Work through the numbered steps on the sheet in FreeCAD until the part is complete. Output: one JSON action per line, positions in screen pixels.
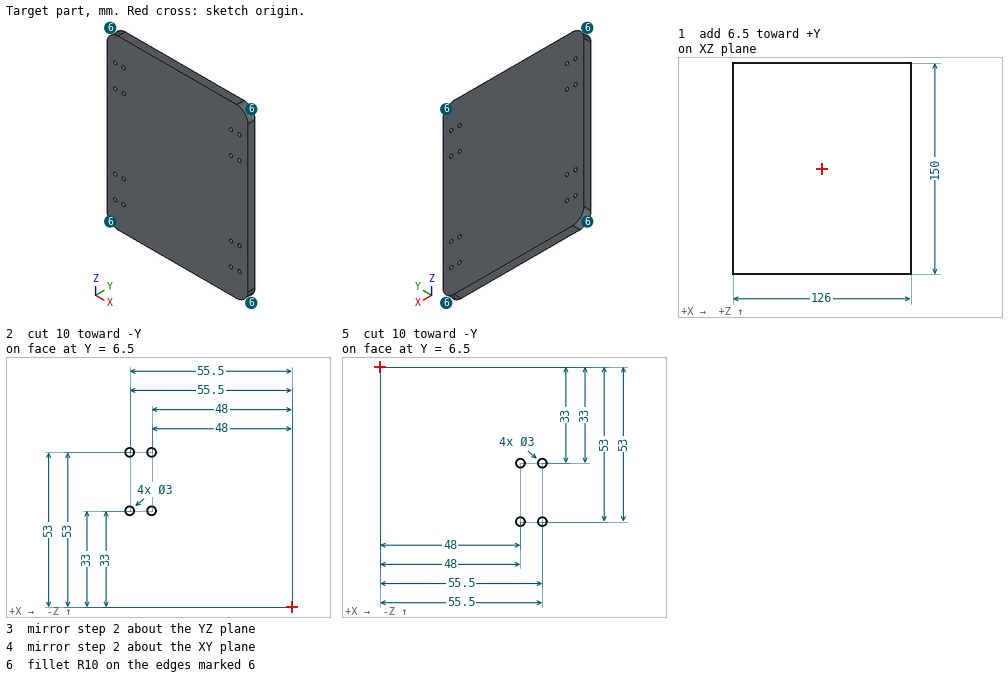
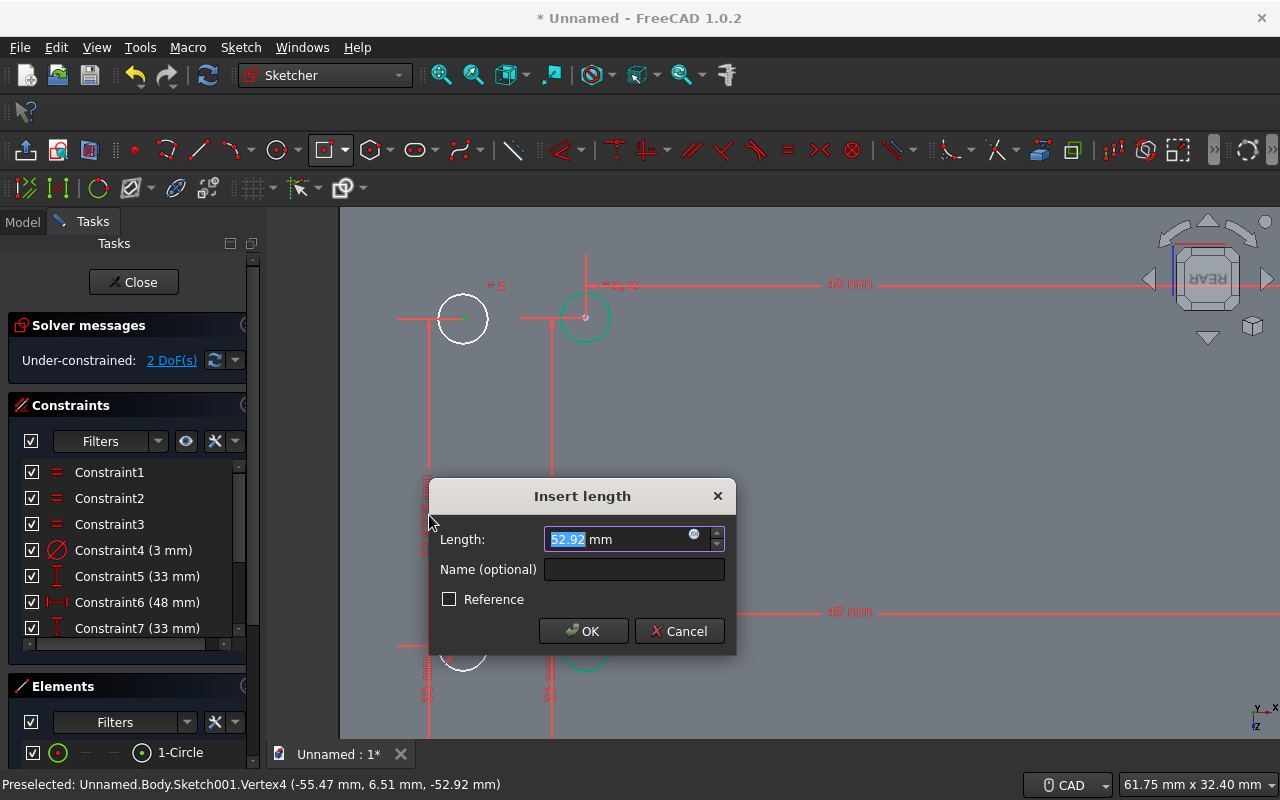
{"action": "type", "text": "53"}
{"action": "key", "text": "Return"}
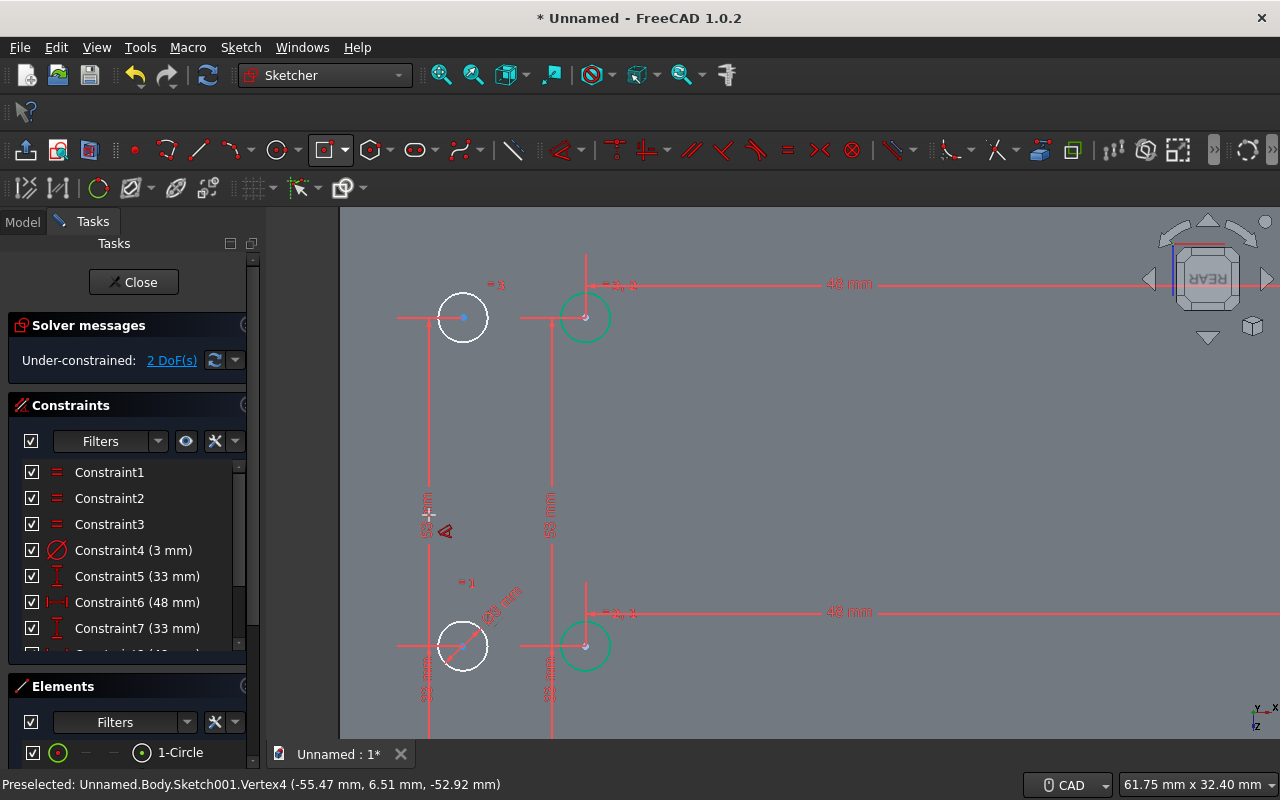
{"action": "left_click", "coordinate": [463, 646]}
{"action": "left_click", "coordinate": [639, 612]}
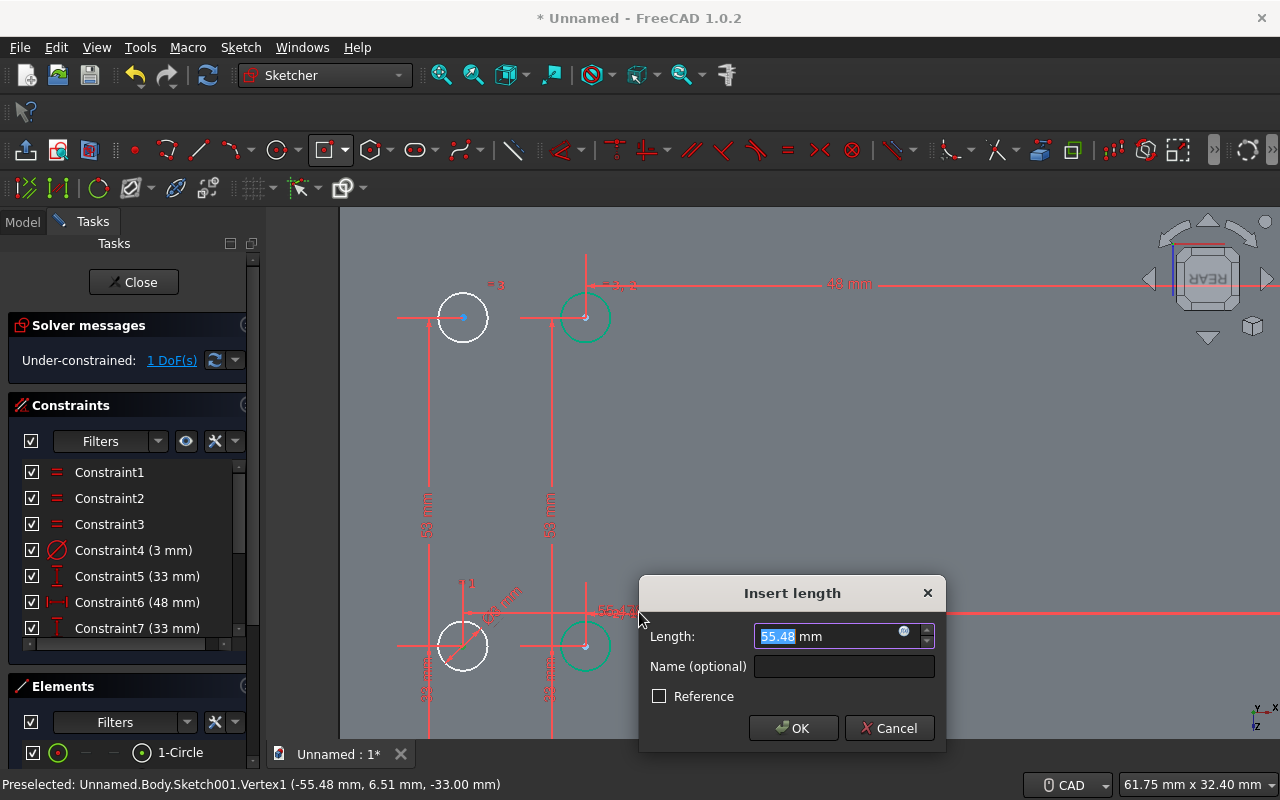
{"action": "type", "text": "55.5"}
{"action": "key", "text": "Return"}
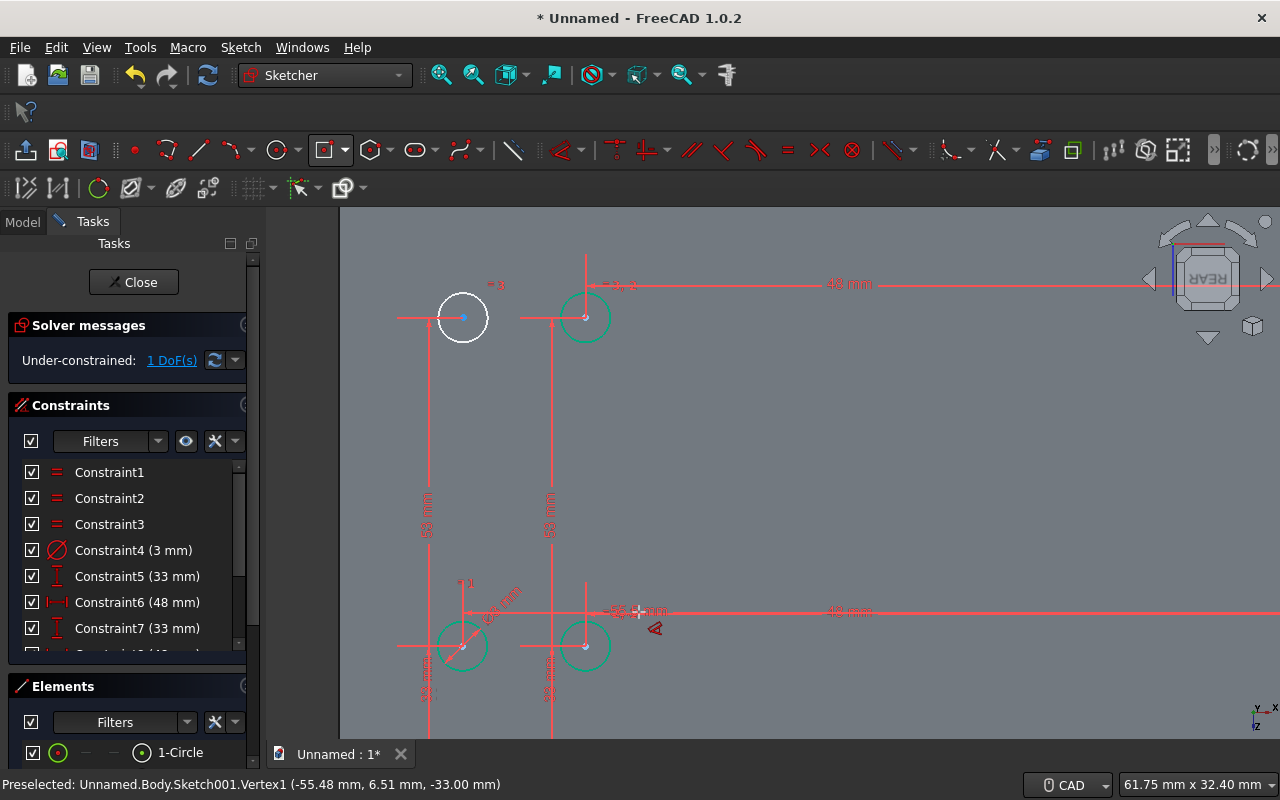
{"action": "left_click", "coordinate": [463, 318]}
{"action": "left_click", "coordinate": [639, 284]}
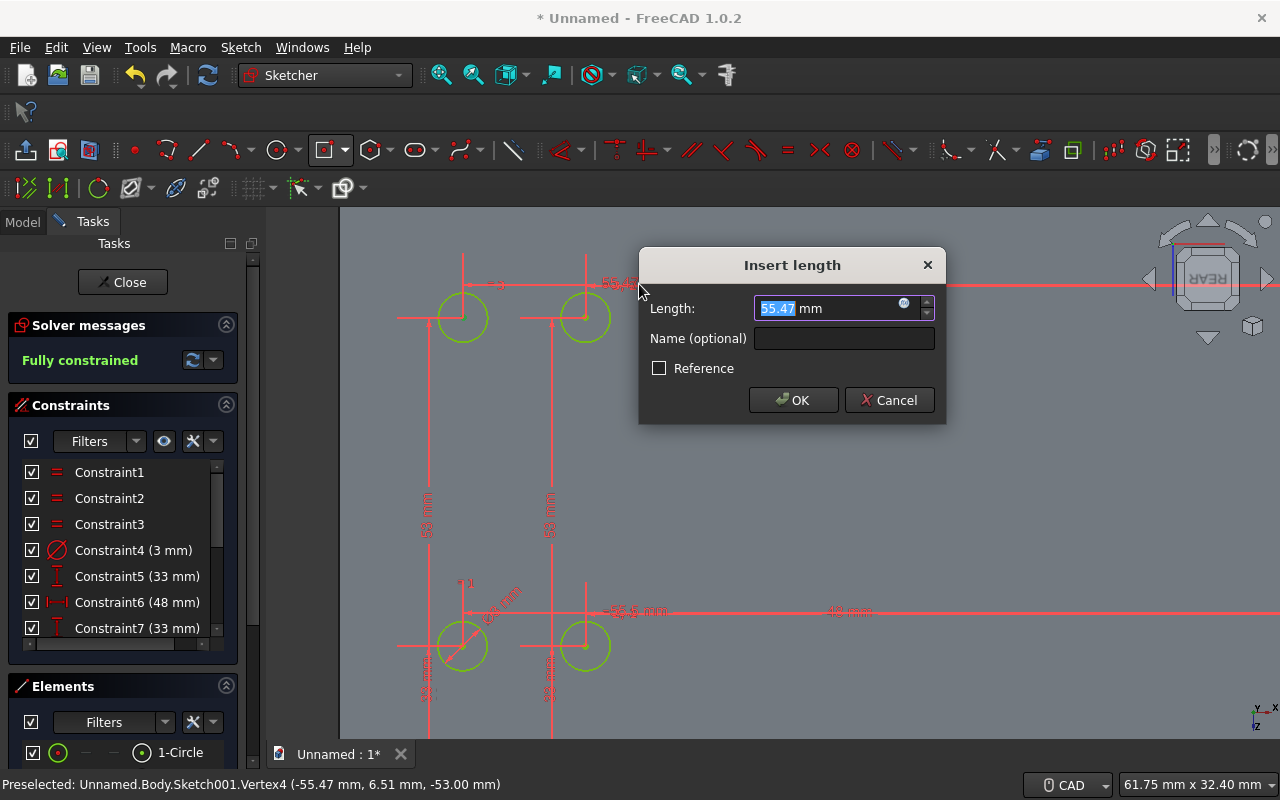
{"action": "type", "text": "55.5"}
{"action": "key", "text": "Return"}
{"action": "key", "text": "Escape"}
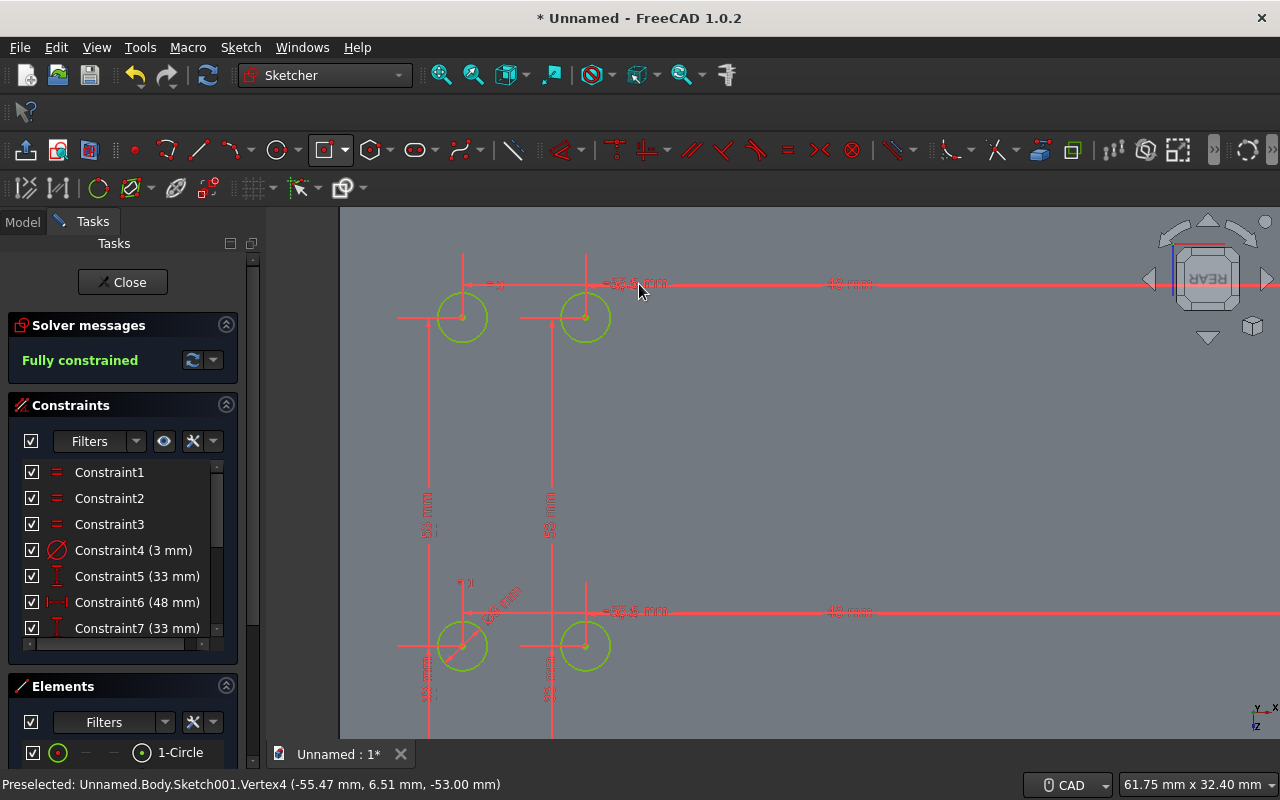
{"action": "left_click", "coordinate": [123, 282]}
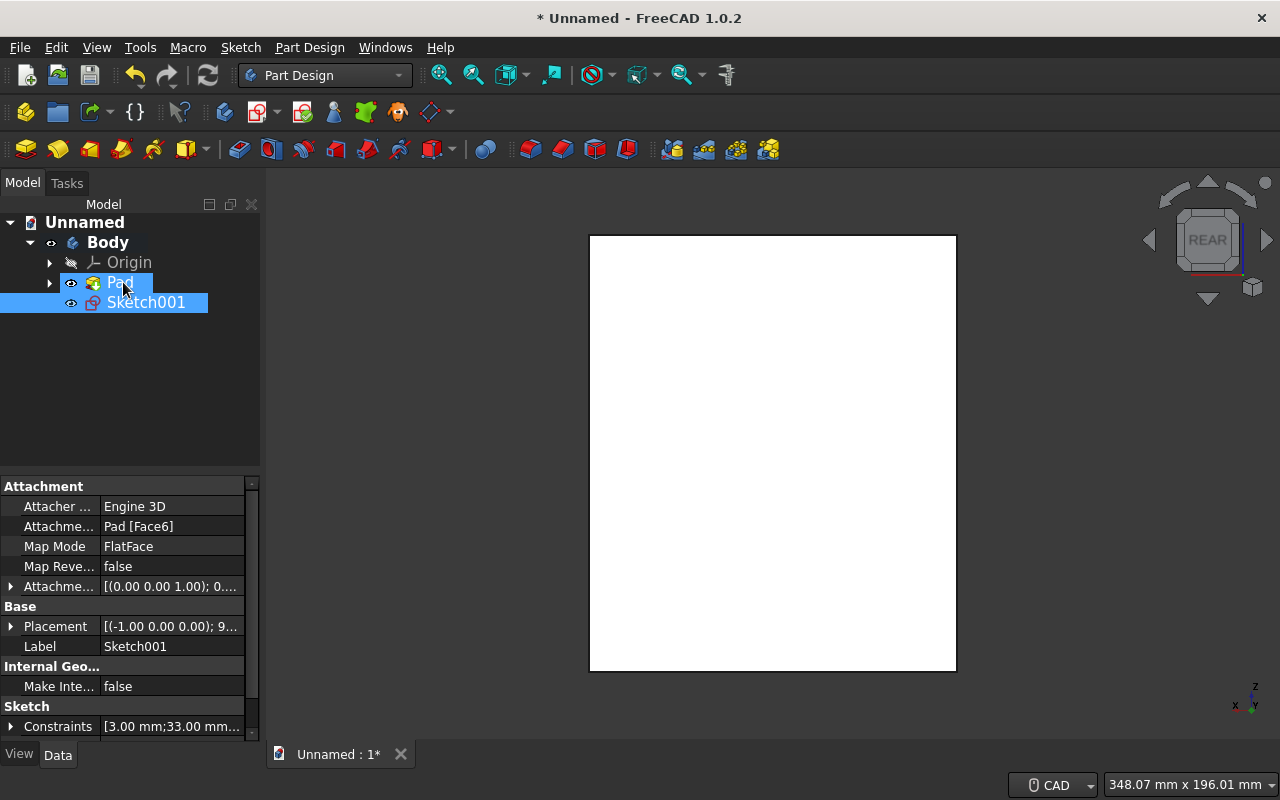
{"action": "left_click", "coordinate": [240, 150]}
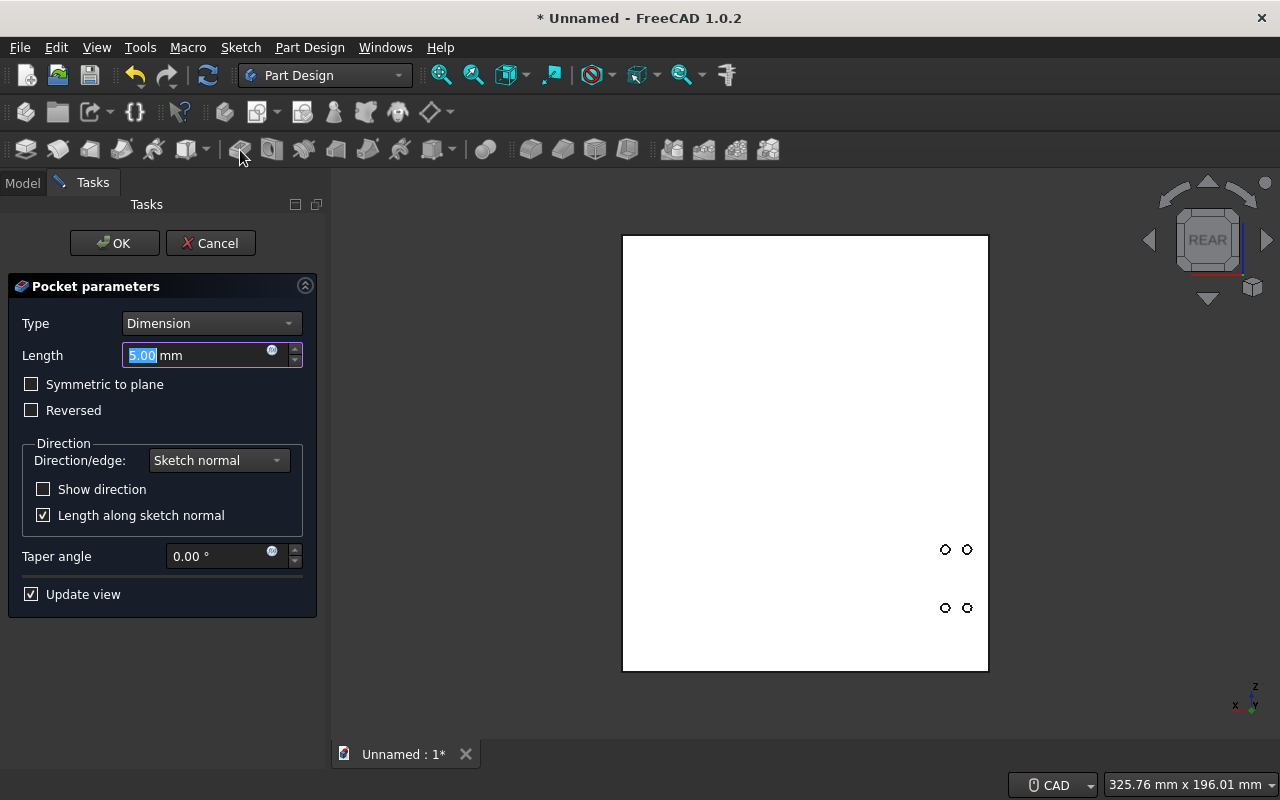
{"action": "type", "text": "10"}
{"action": "key", "text": "Tab"}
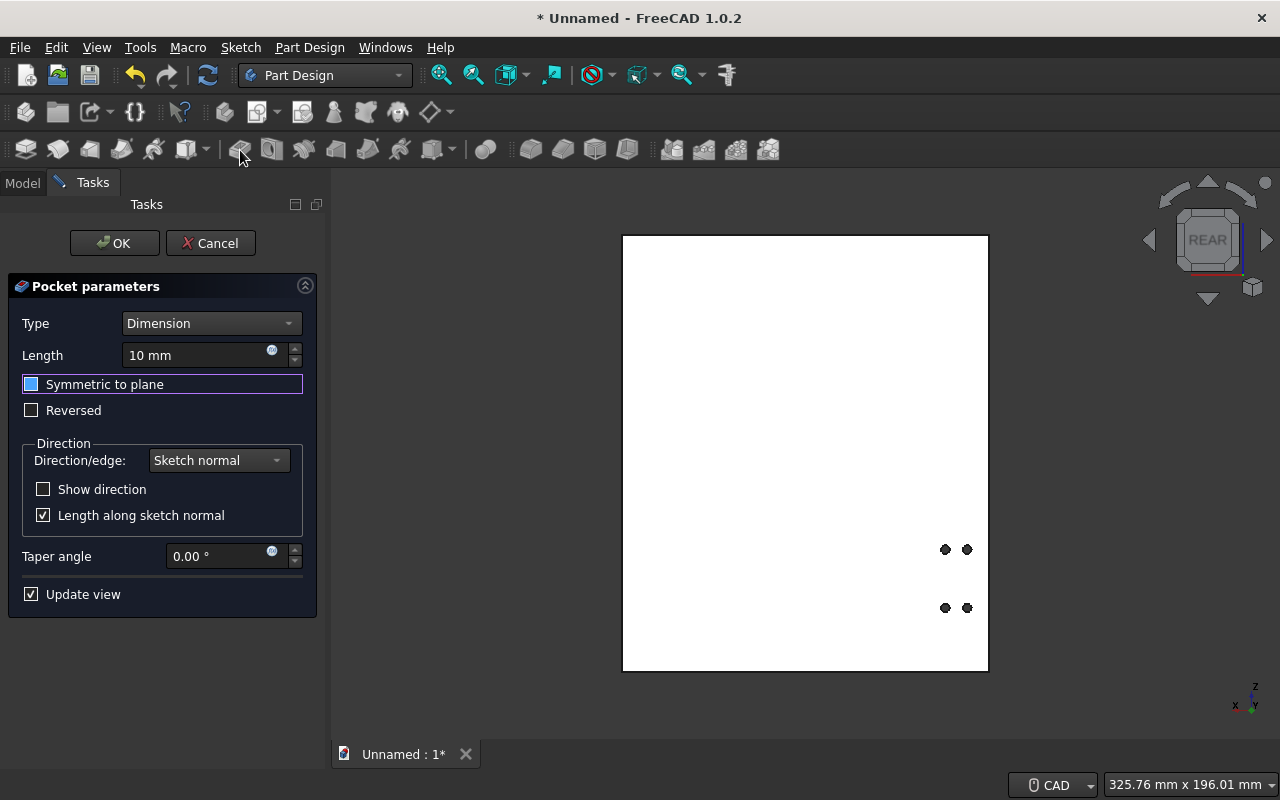
{"action": "left_click", "coordinate": [115, 243]}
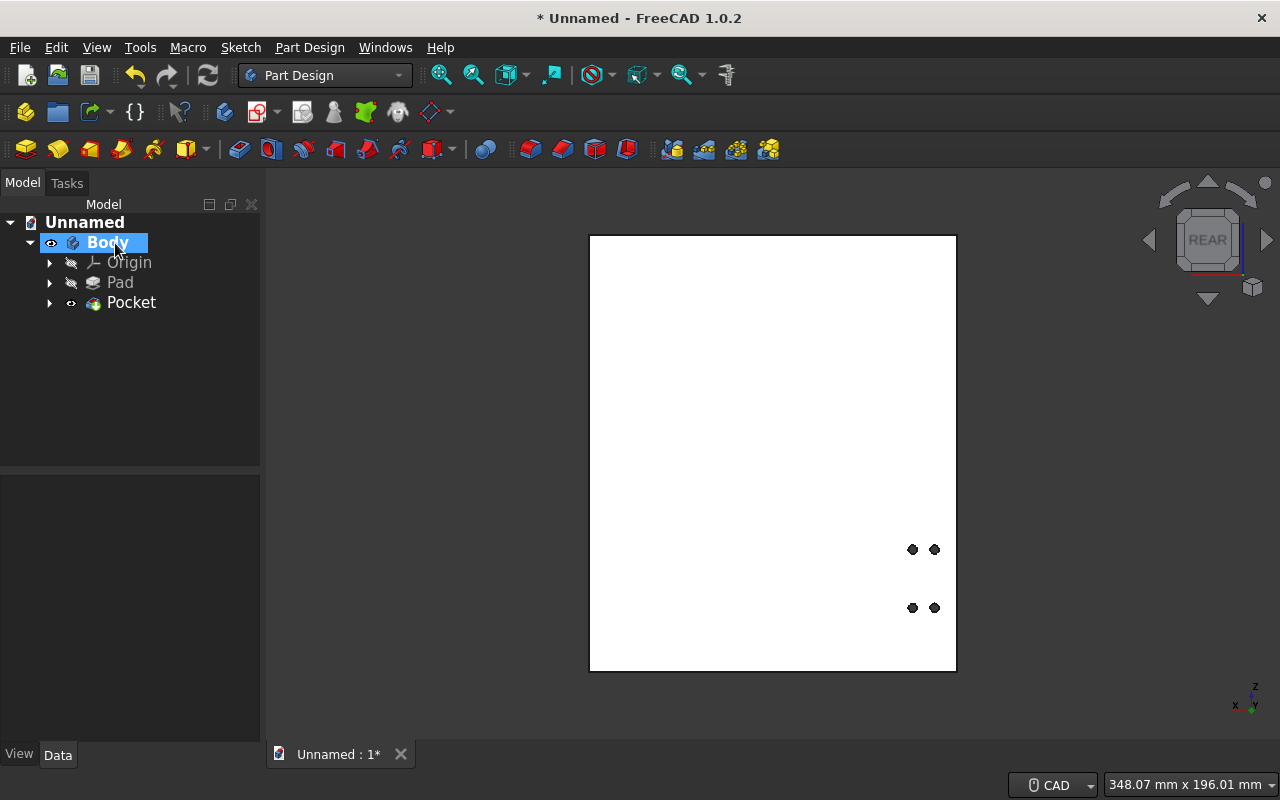
{"action": "left_click", "coordinate": [116, 303]}